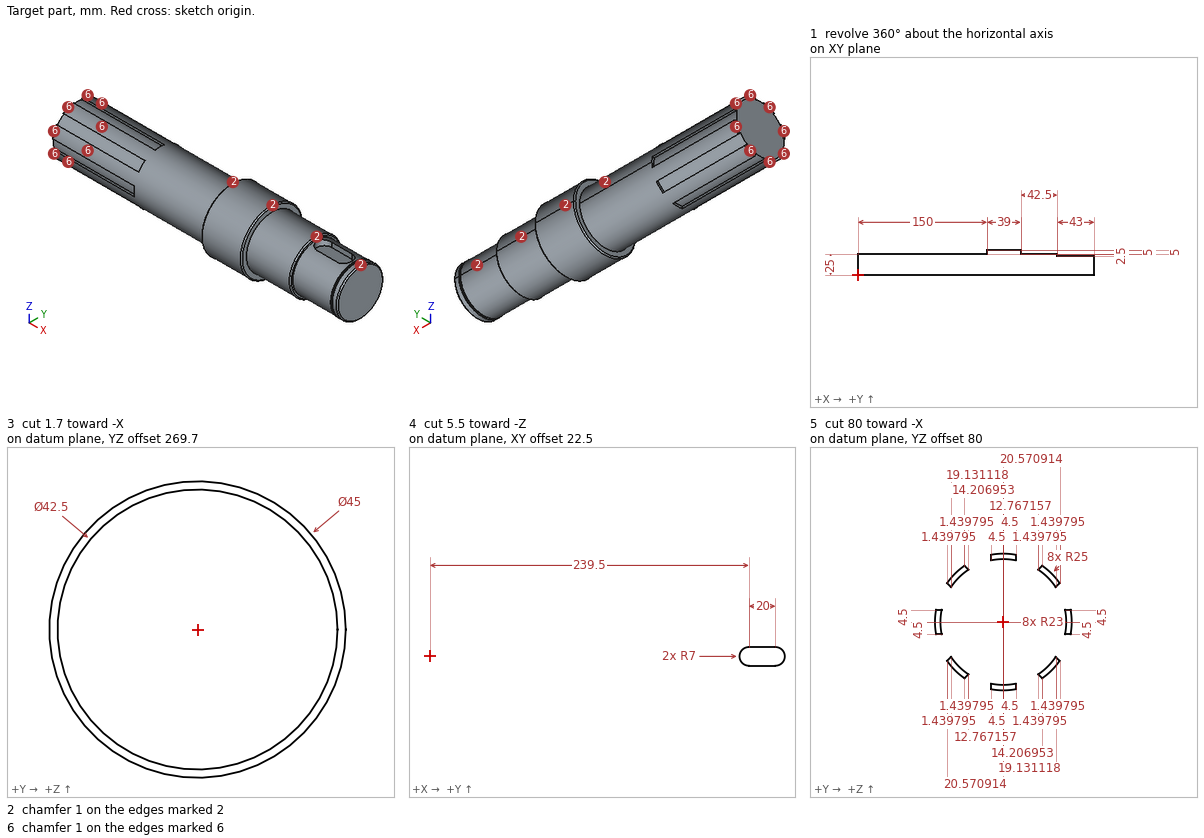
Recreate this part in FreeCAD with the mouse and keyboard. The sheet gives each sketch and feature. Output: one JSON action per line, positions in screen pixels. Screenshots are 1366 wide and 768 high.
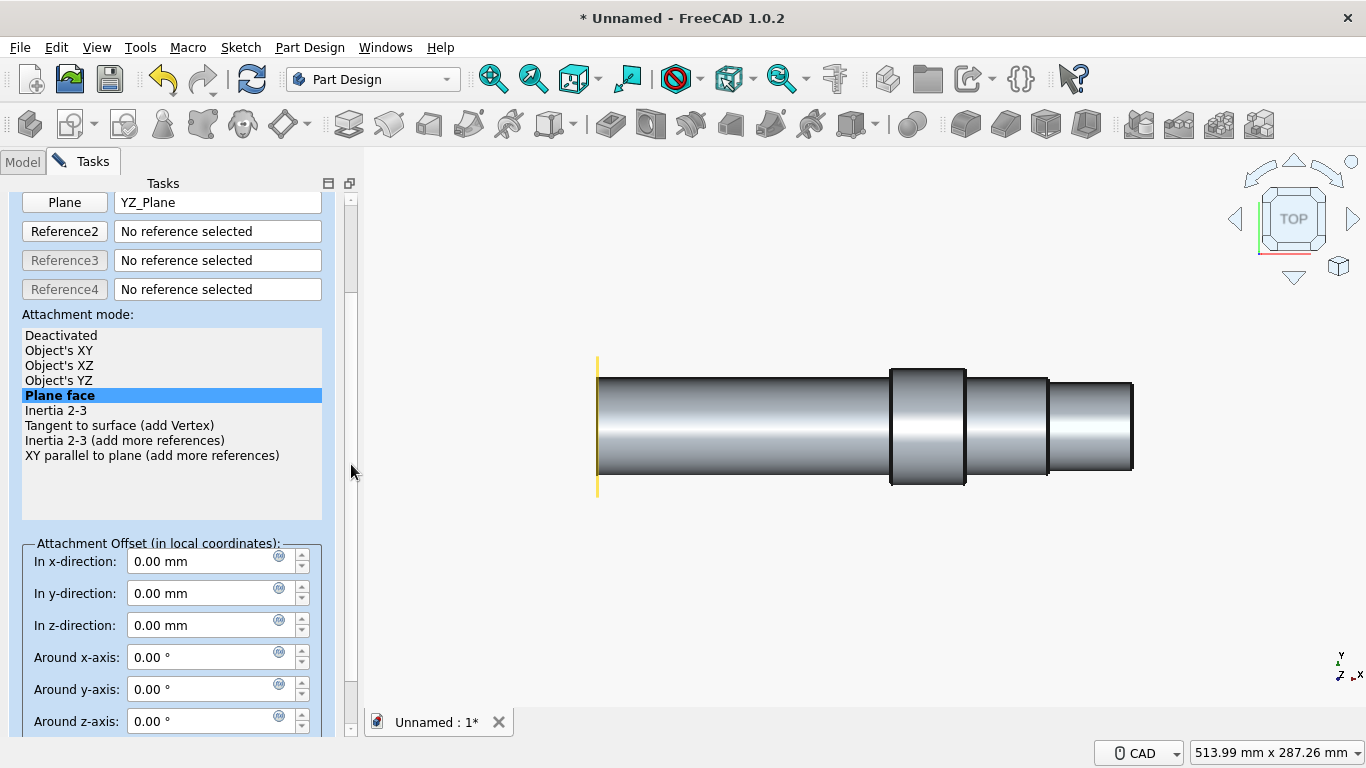
{"action": "triple_click", "coordinate": [210, 625]}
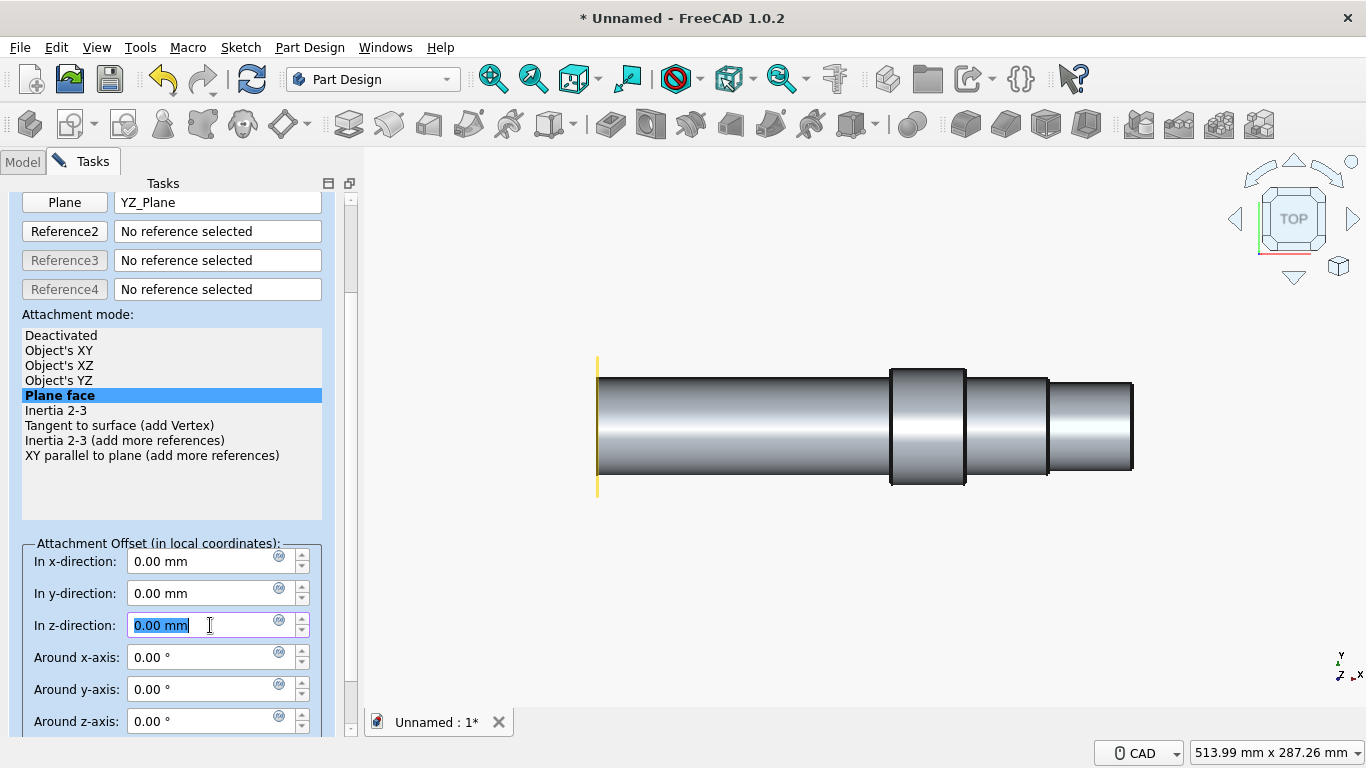
{"action": "type", "text": "269.7"}
{"action": "key", "text": "Tab"}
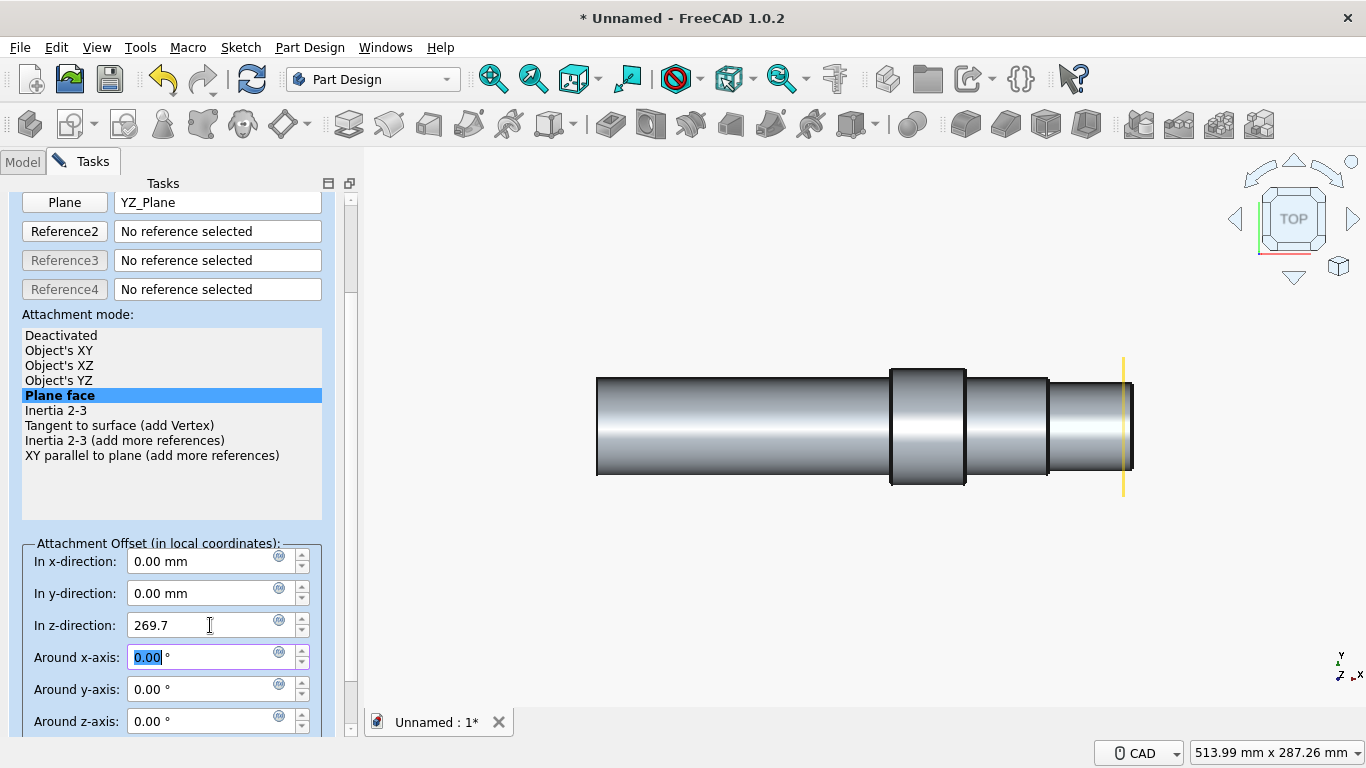
{"action": "scroll", "coordinate": [351, 464], "scroll_direction": "up", "scroll_amount": 3}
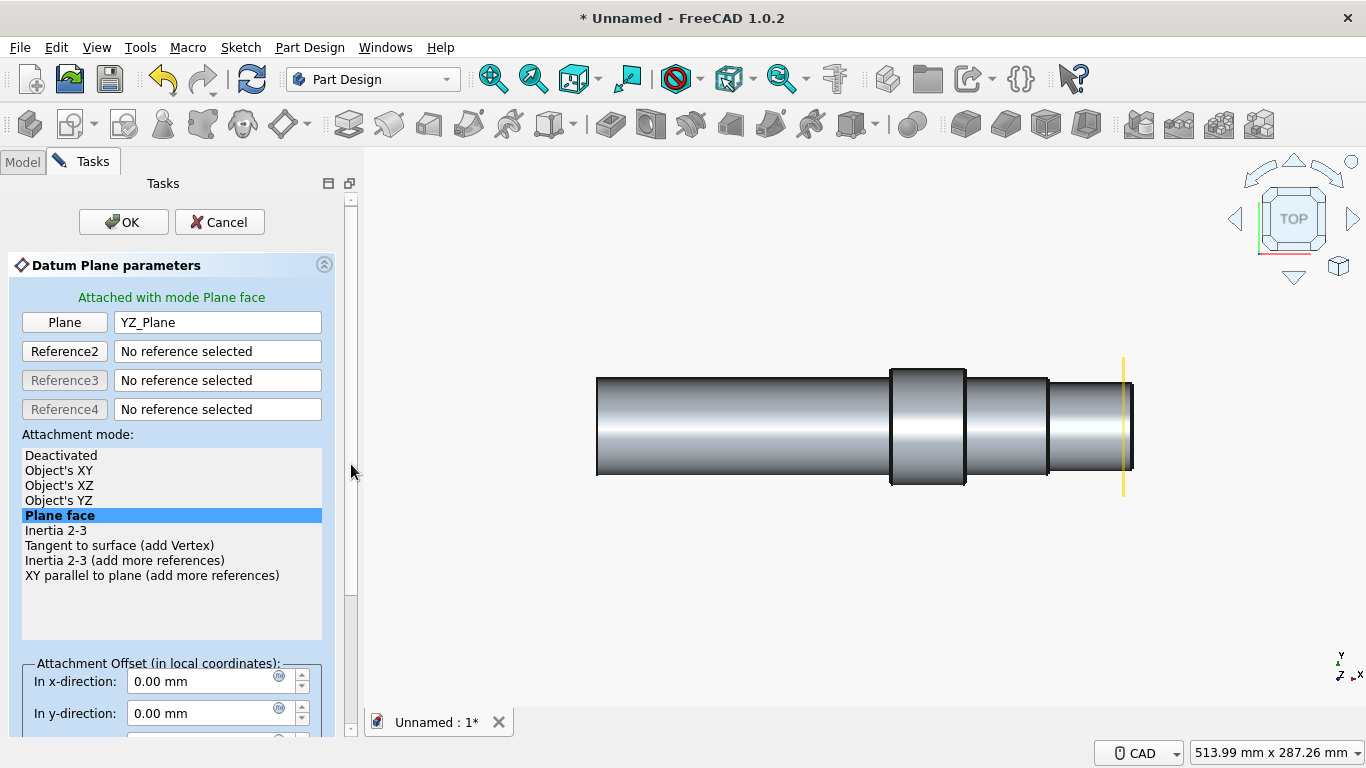
{"action": "left_click", "coordinate": [124, 222]}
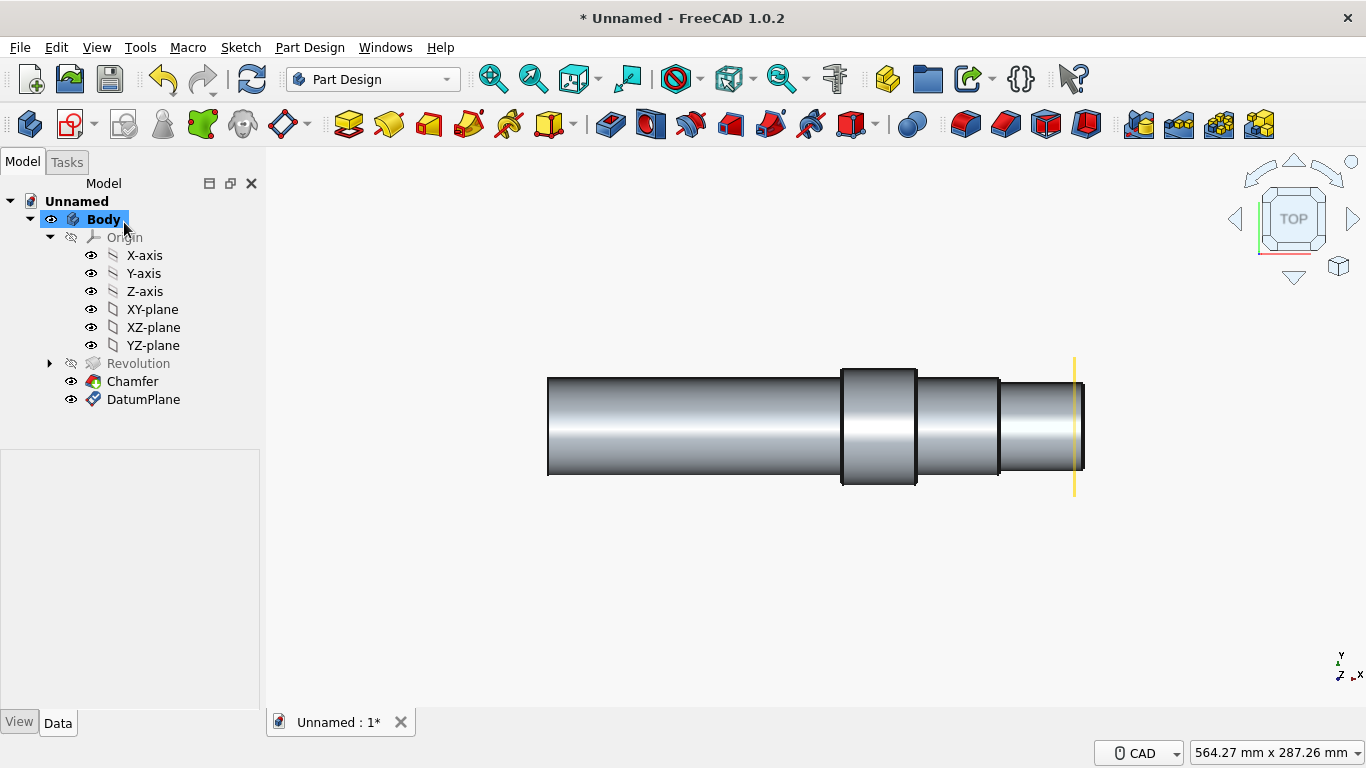
{"action": "left_click", "coordinate": [116, 399]}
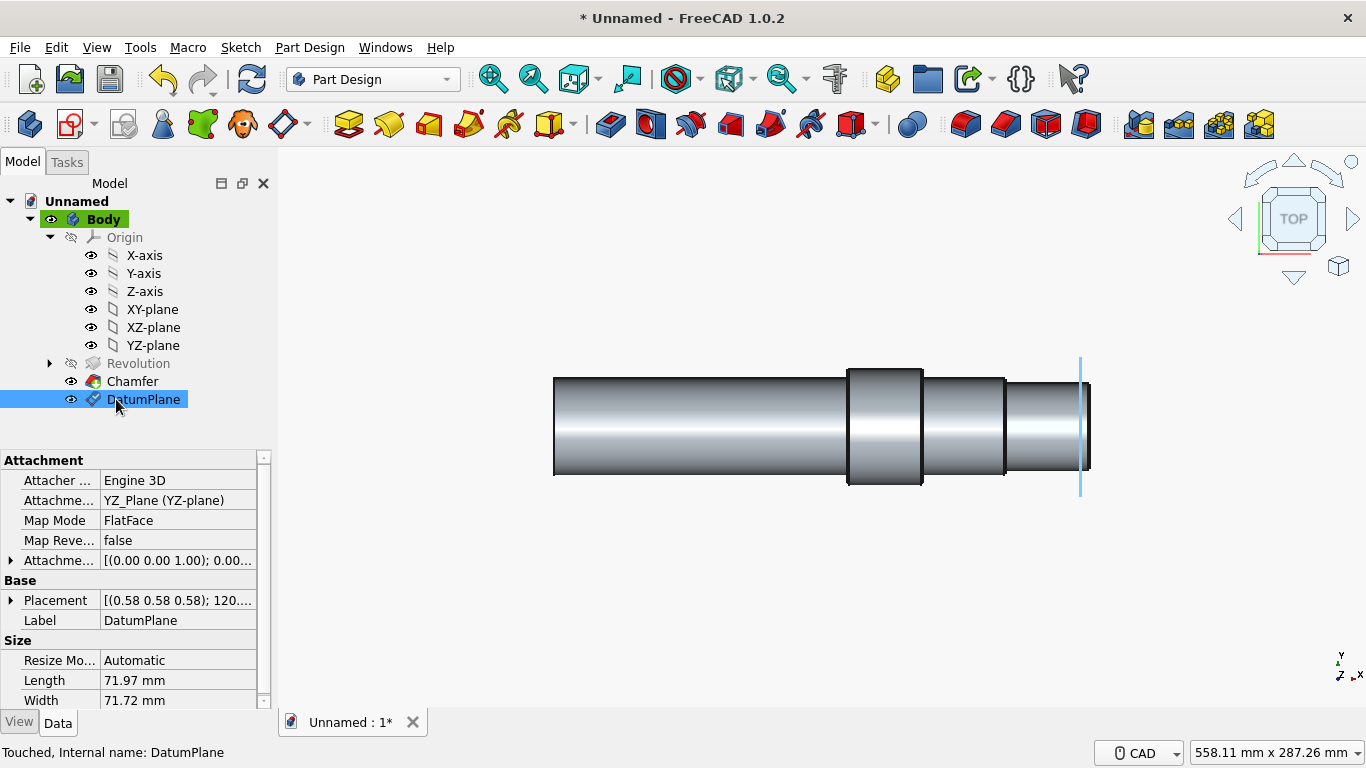
{"action": "left_click", "coordinate": [70, 124]}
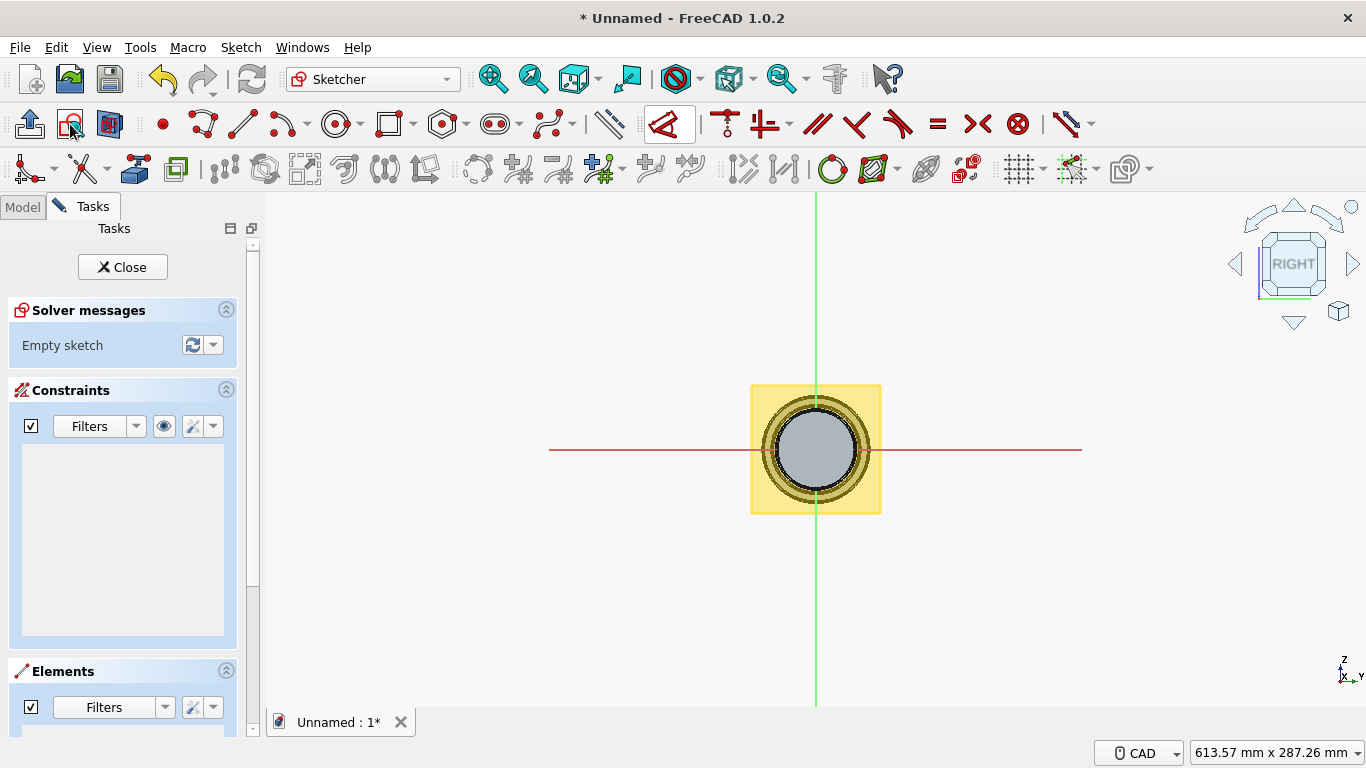
{"action": "left_click", "coordinate": [110, 124]}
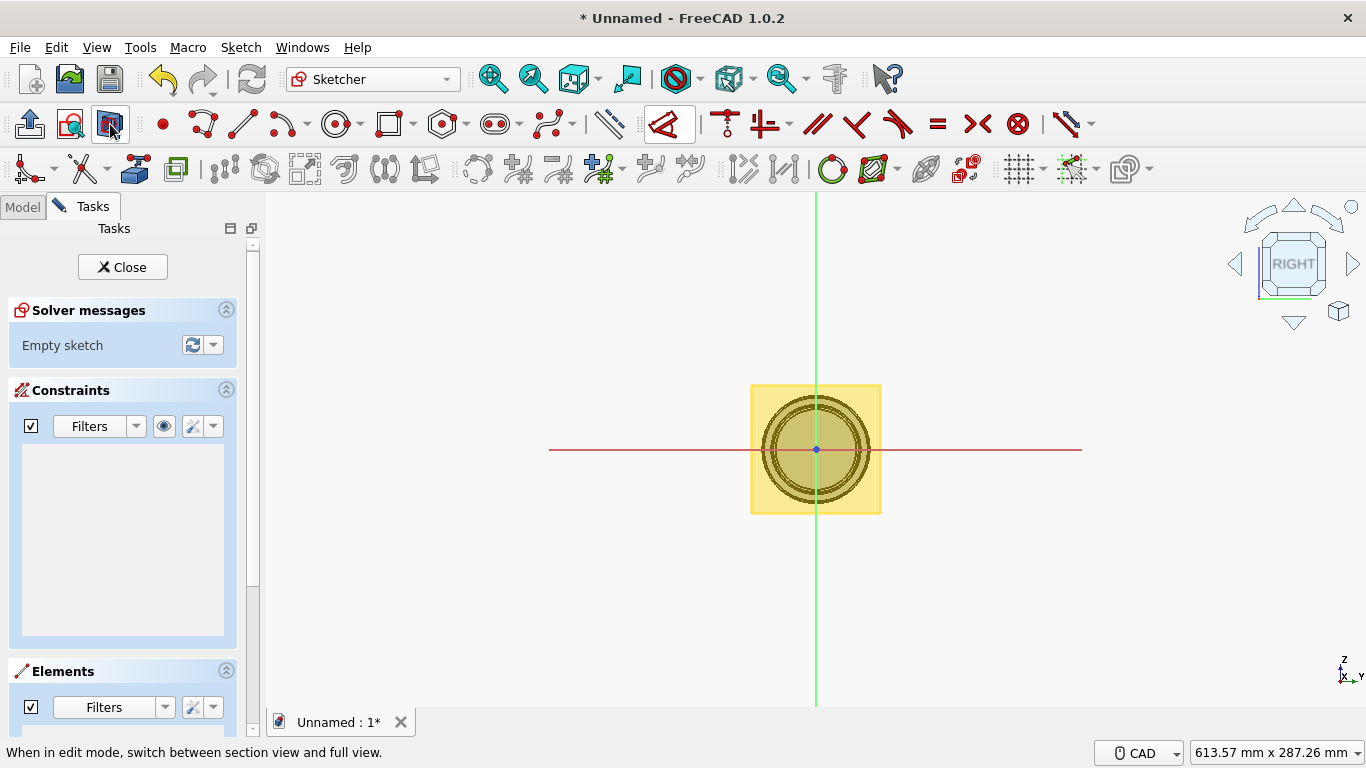
{"action": "scroll", "coordinate": [838, 449], "scroll_direction": "up", "scroll_amount": 7}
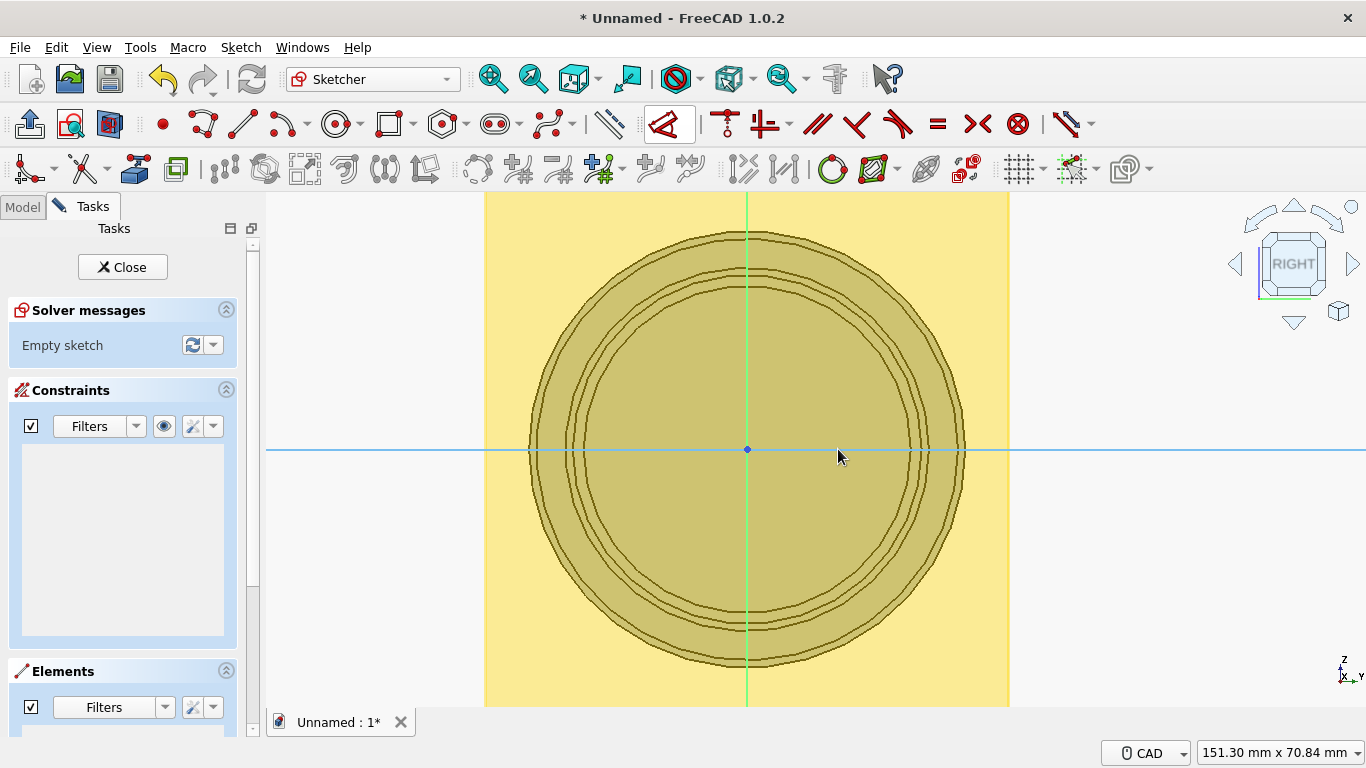
{"action": "left_click", "coordinate": [336, 124]}